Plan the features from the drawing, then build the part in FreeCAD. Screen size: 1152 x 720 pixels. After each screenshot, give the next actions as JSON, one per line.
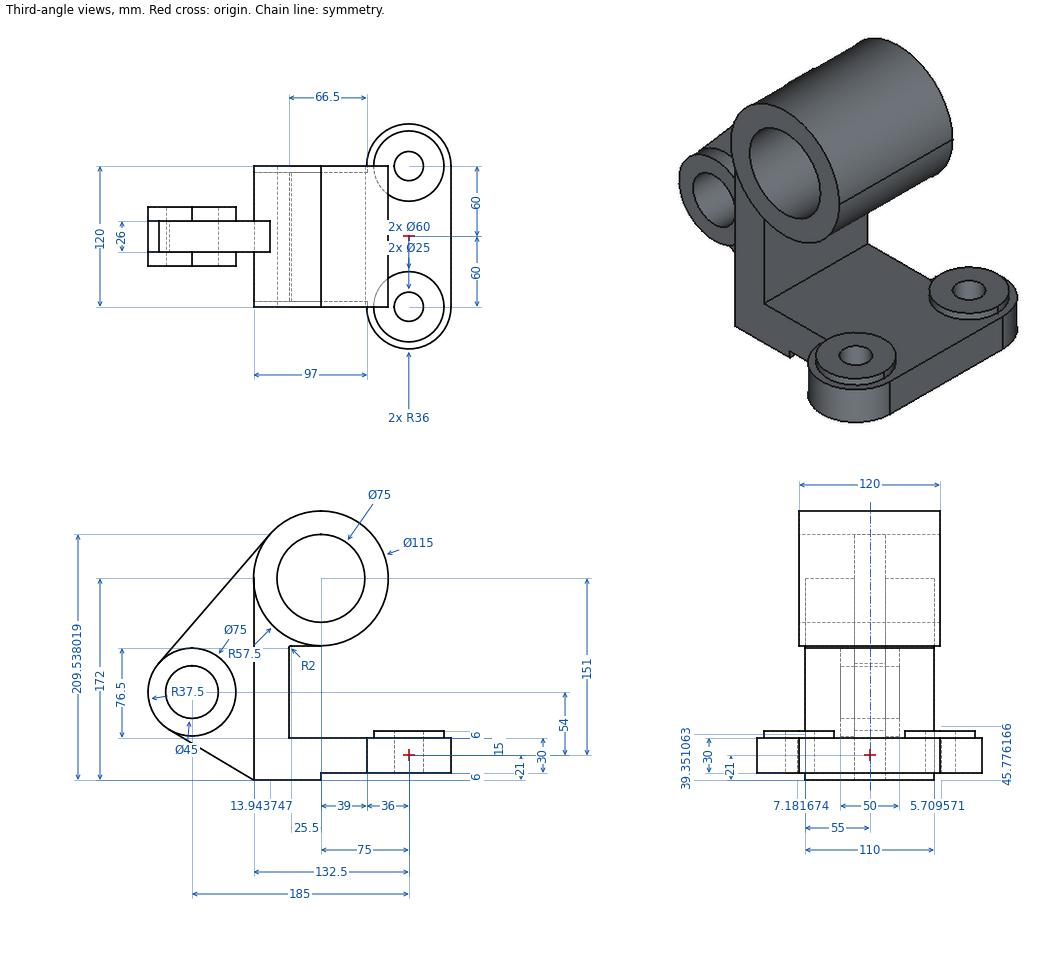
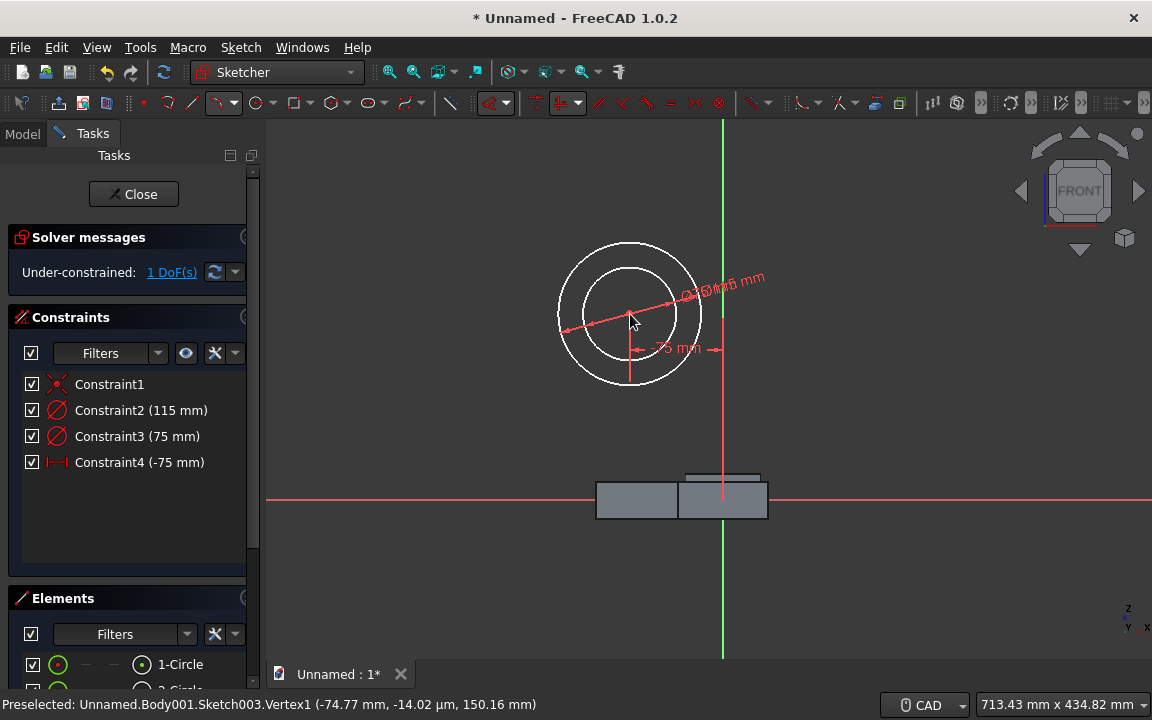
{"action": "left_click", "coordinate": [630, 314]}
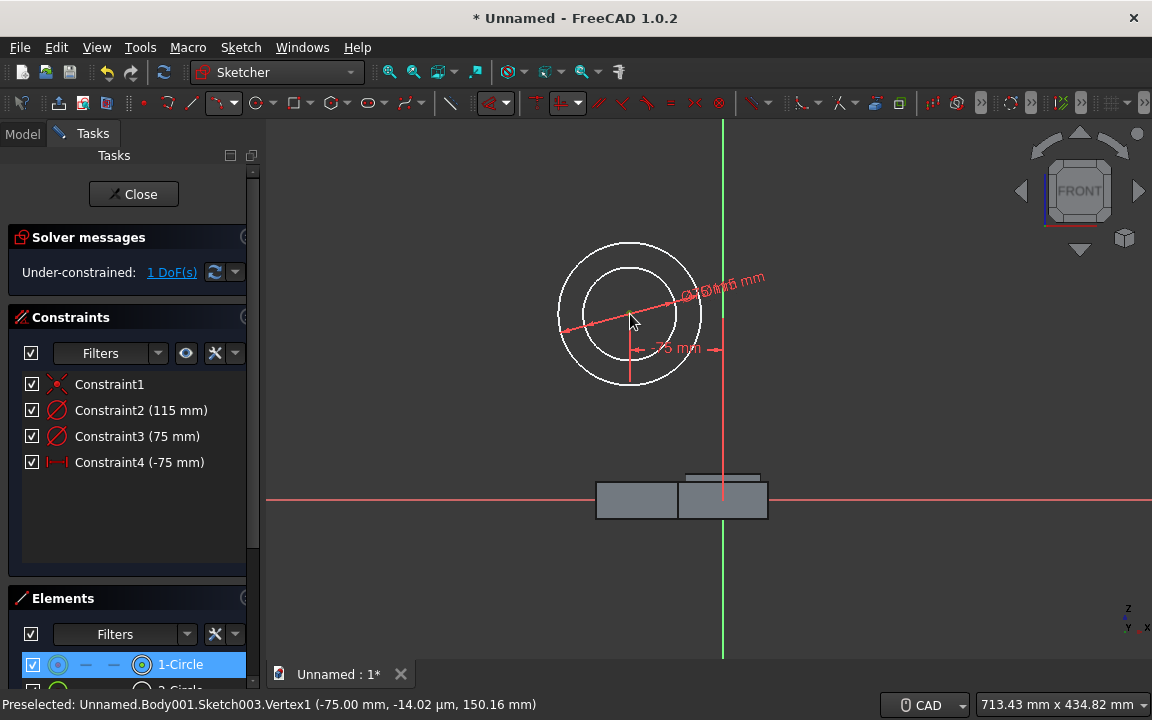
{"action": "key", "text": "i"}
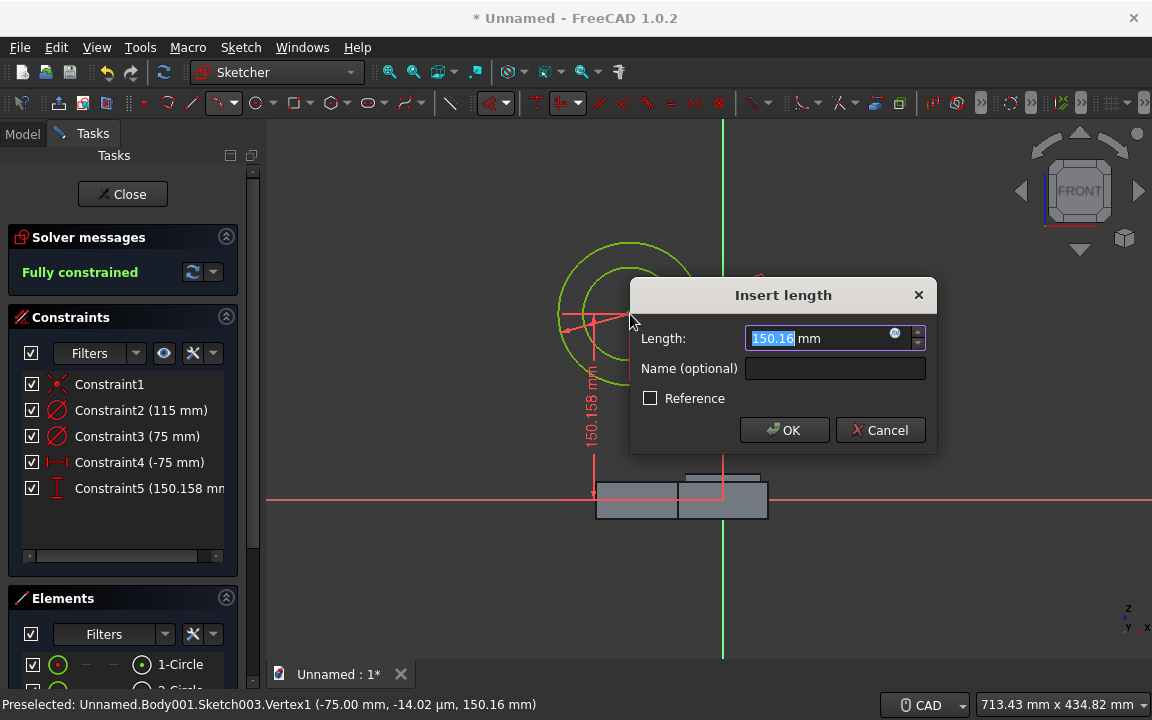
{"action": "type", "text": "151"}
{"action": "key", "text": "Return"}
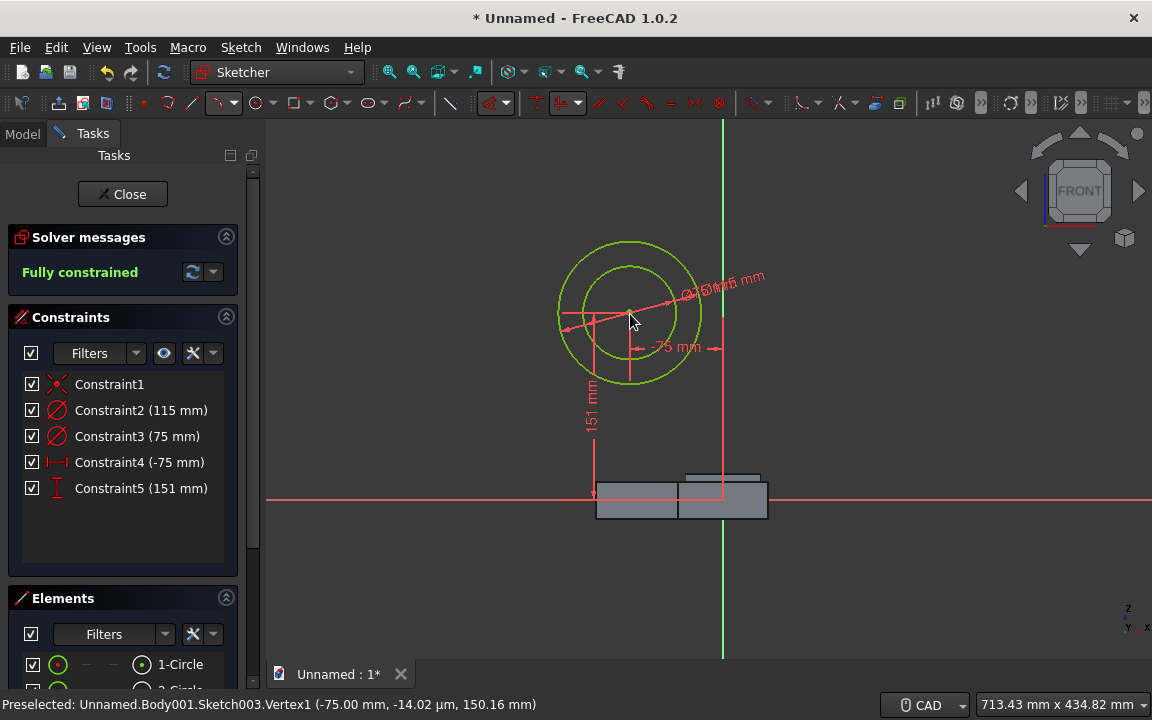
{"action": "left_click", "coordinate": [123, 194]}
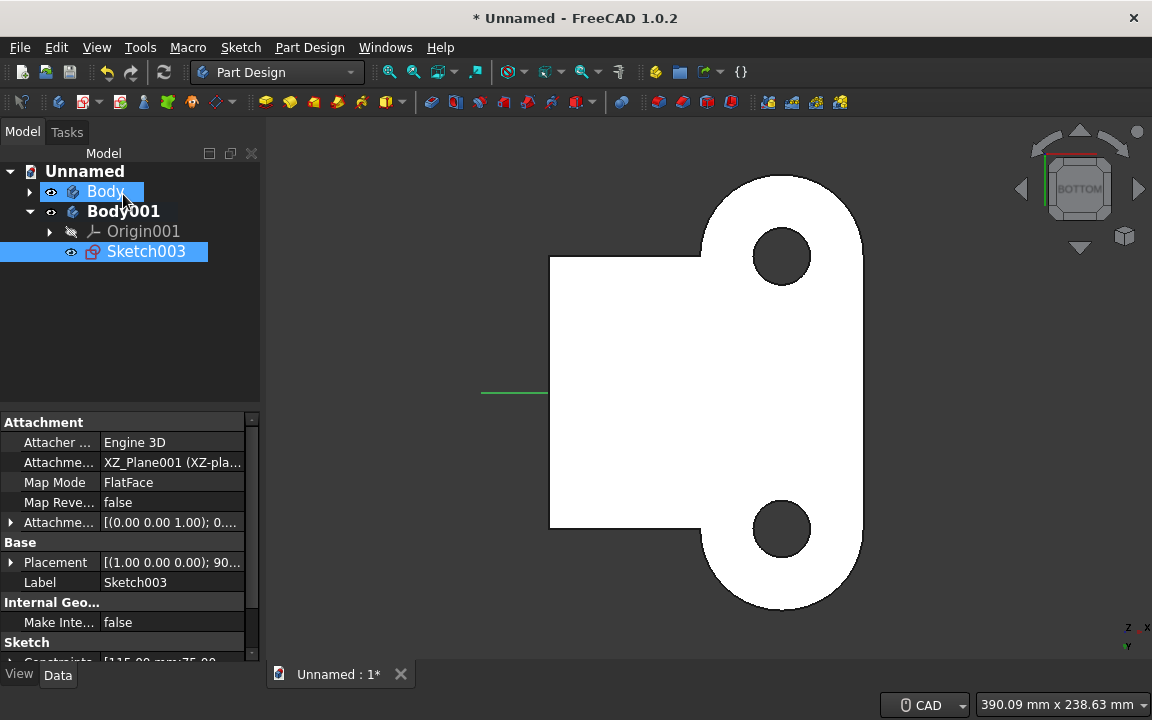
{"action": "left_click", "coordinate": [266, 102]}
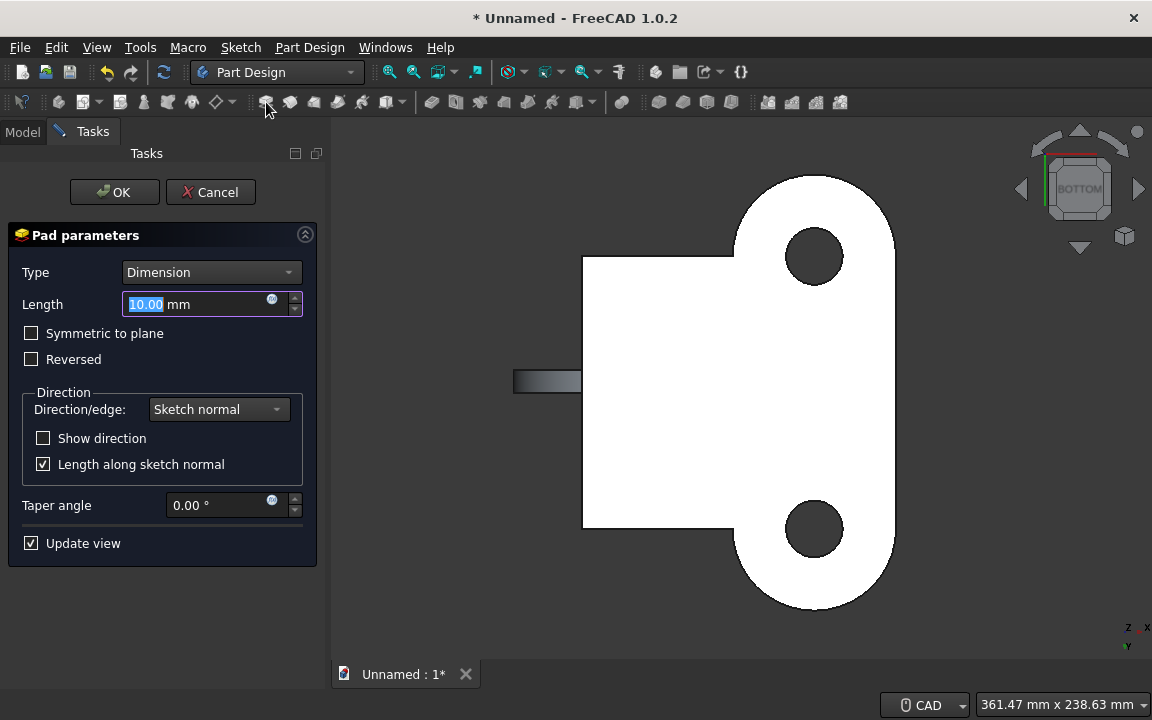
{"action": "type", "text": "120"}
{"action": "key", "text": "Tab"}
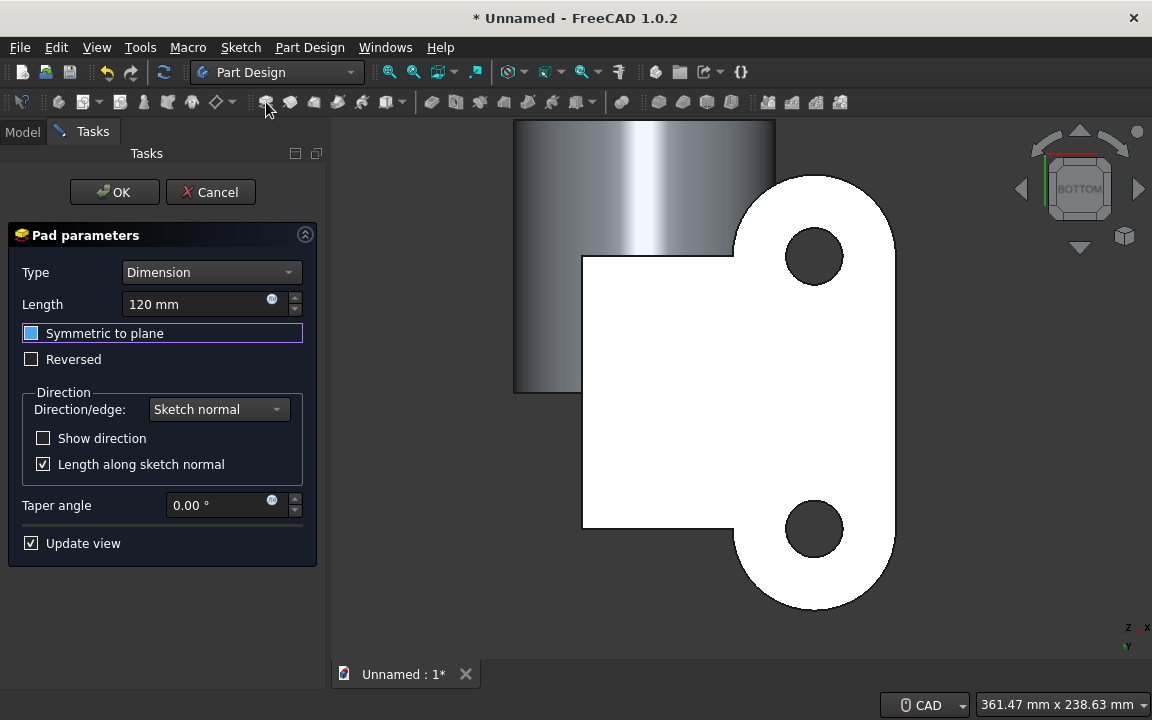
{"action": "left_click", "coordinate": [30, 333]}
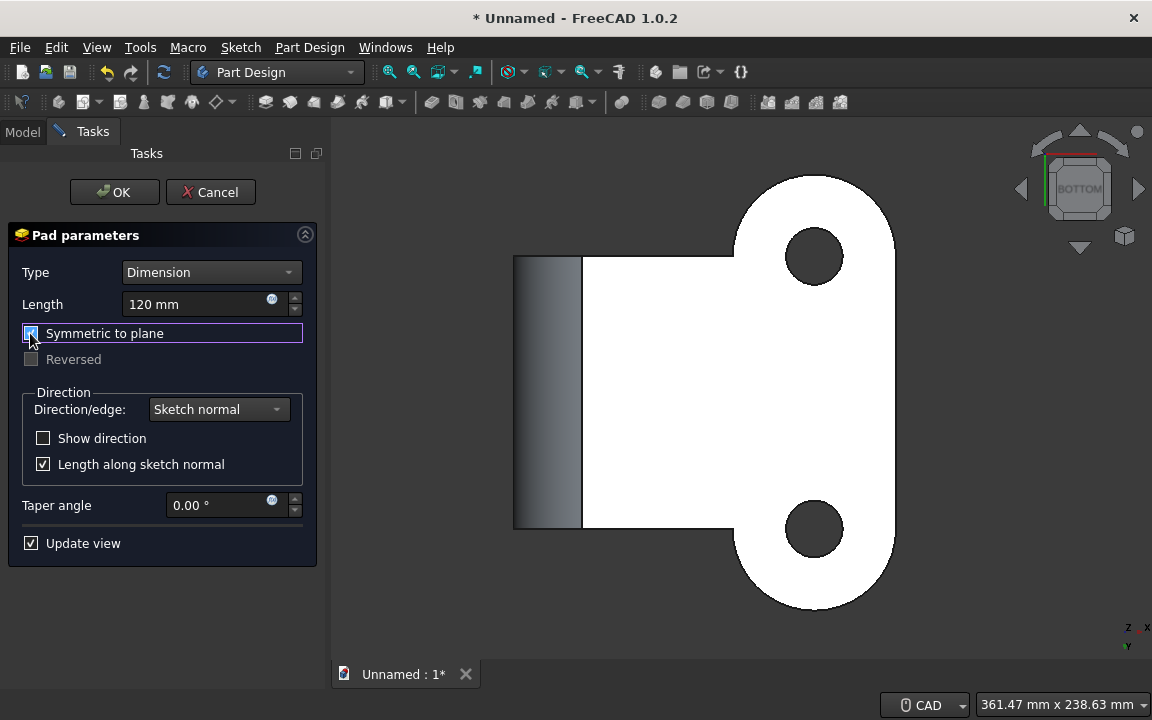
{"action": "left_click", "coordinate": [115, 192]}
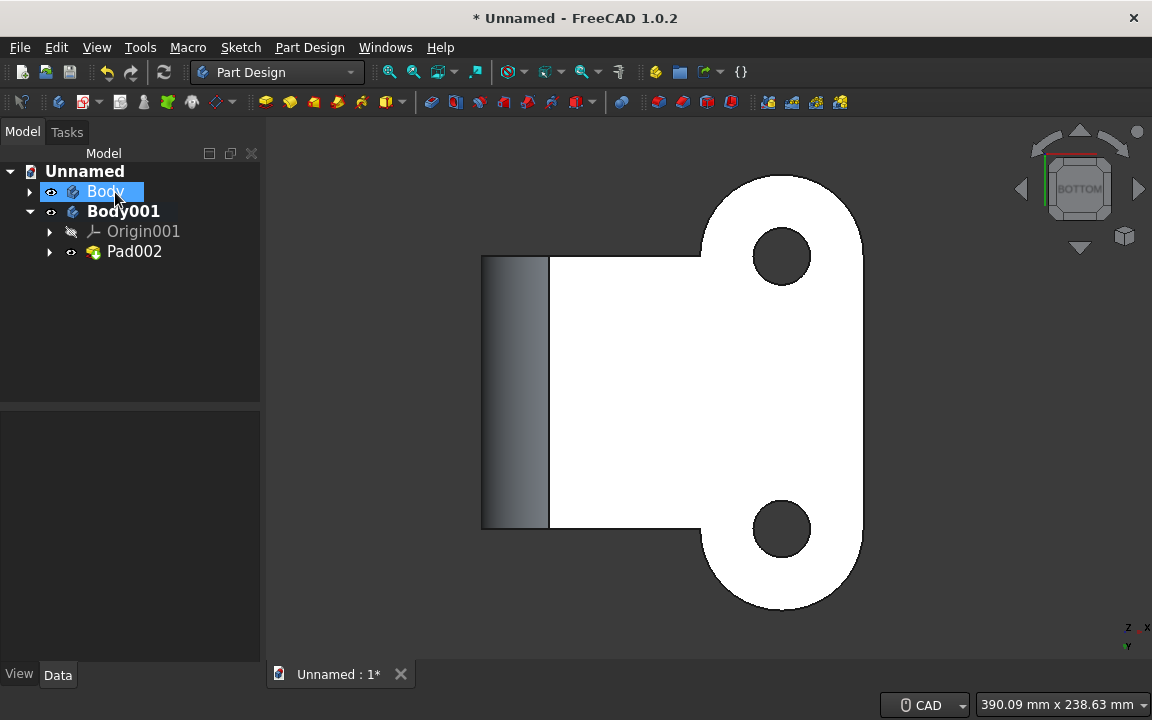
{"action": "double_click", "coordinate": [96, 192]}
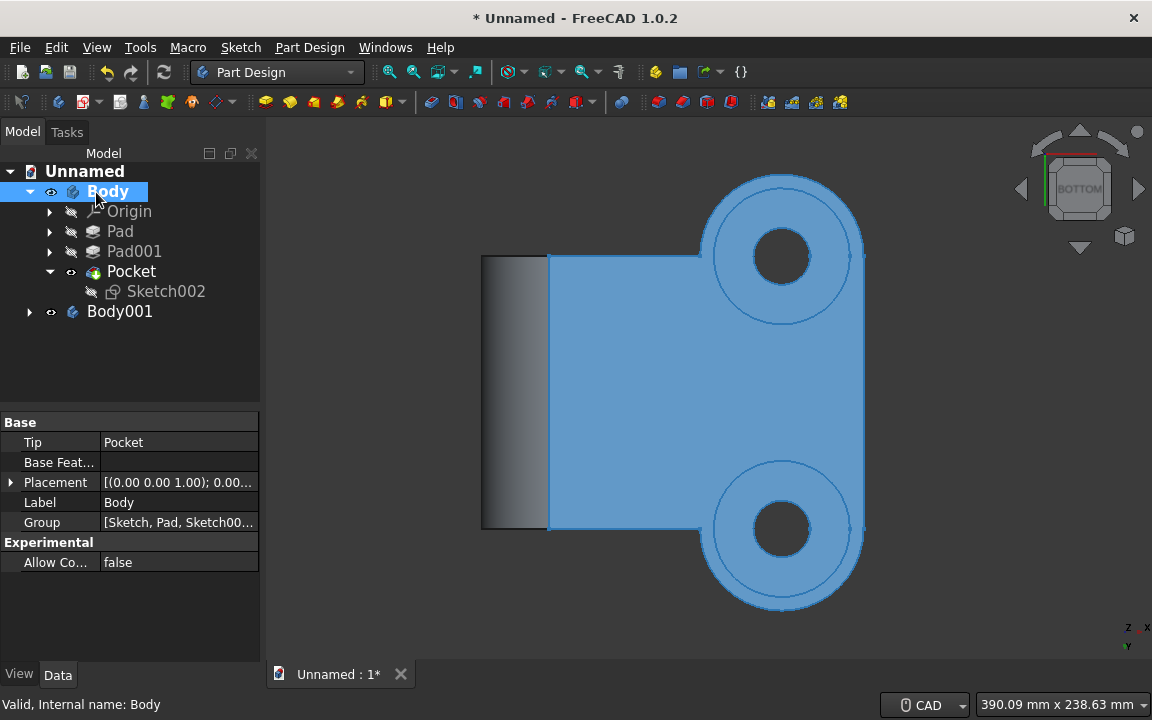
{"action": "left_click", "coordinate": [96, 192]}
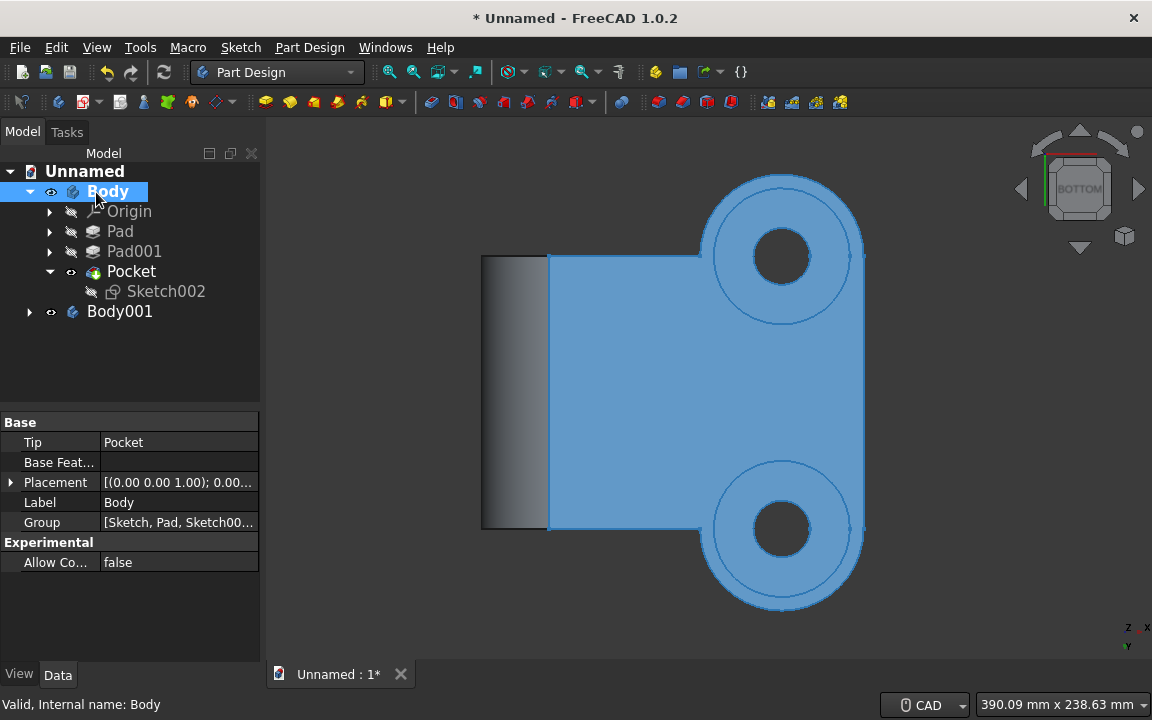
{"action": "left_click", "coordinate": [146, 562]}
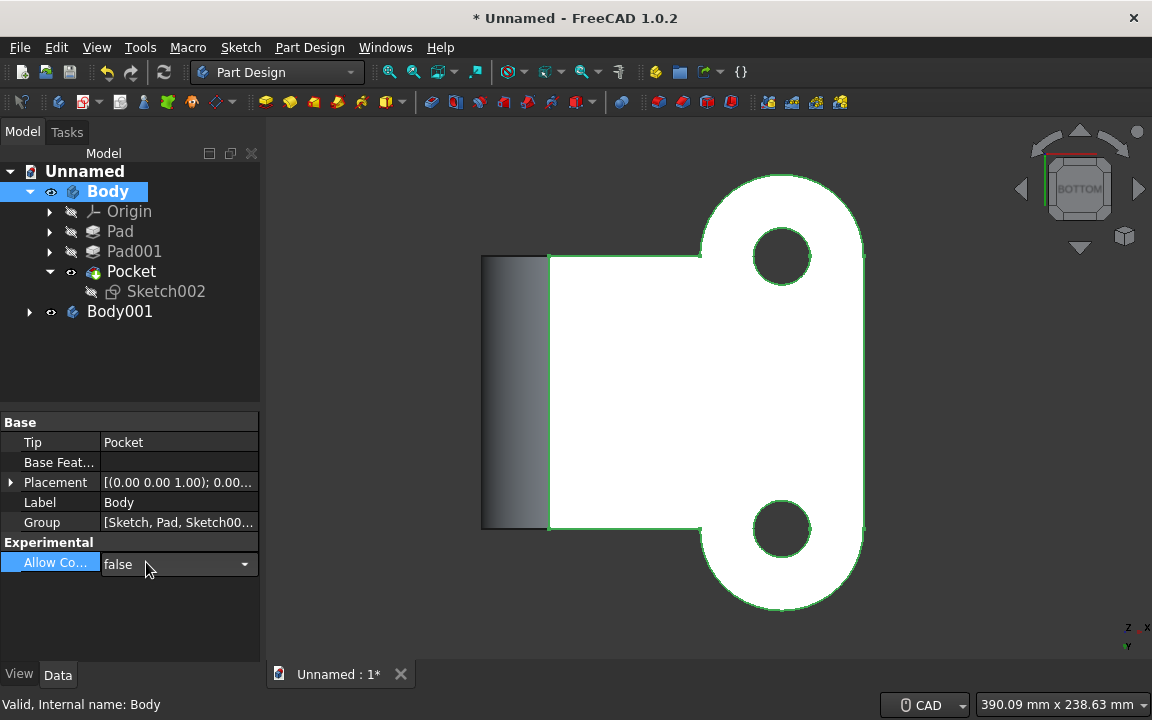
{"action": "left_click", "coordinate": [146, 562]}